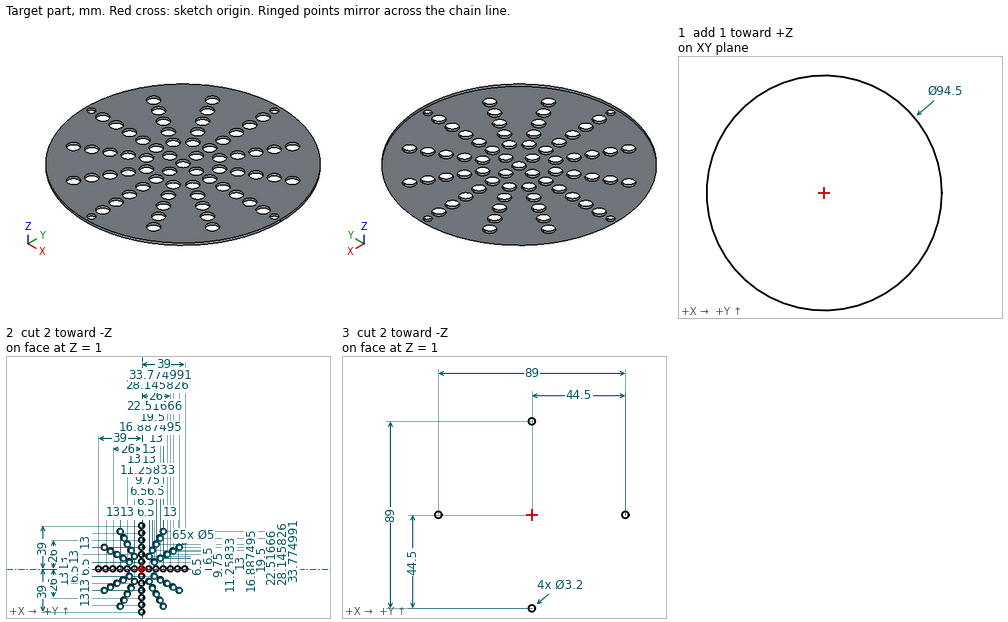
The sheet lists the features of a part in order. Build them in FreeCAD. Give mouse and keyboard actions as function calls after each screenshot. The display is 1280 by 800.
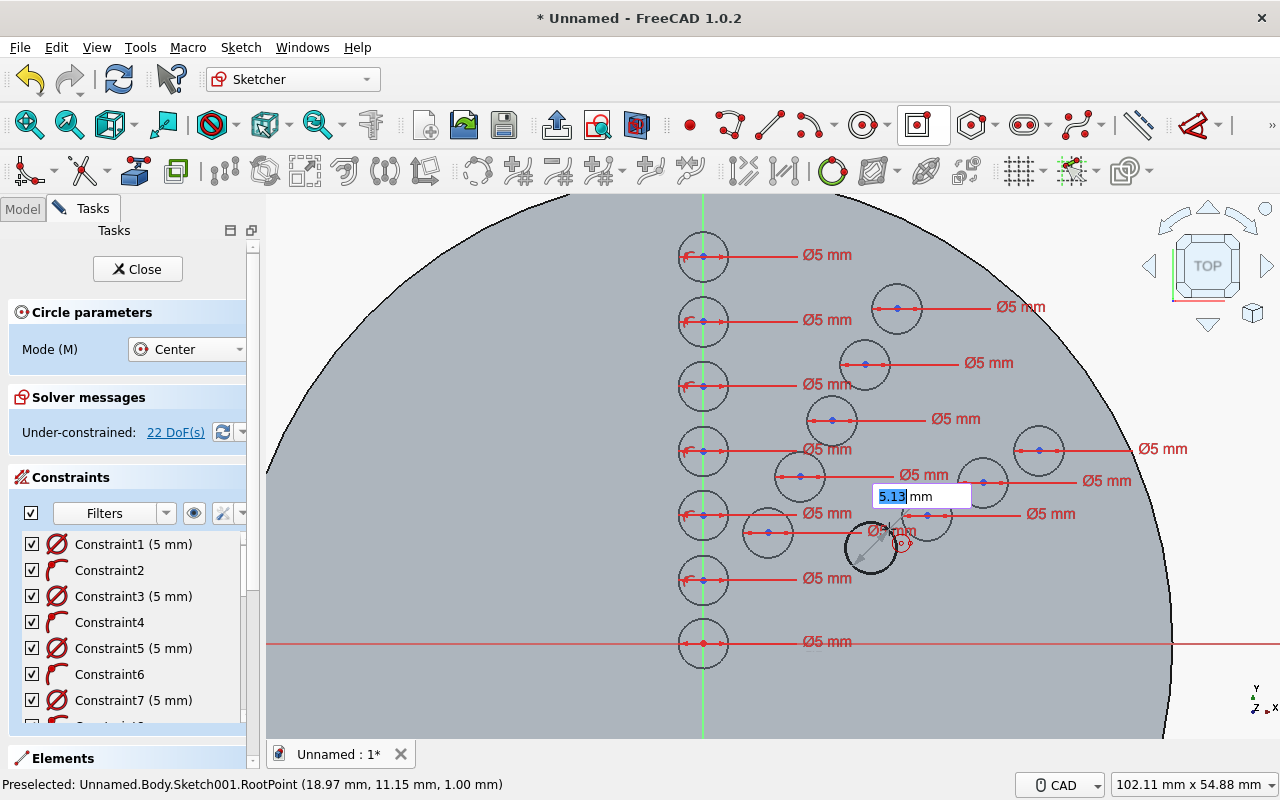
text(5)
key(Return)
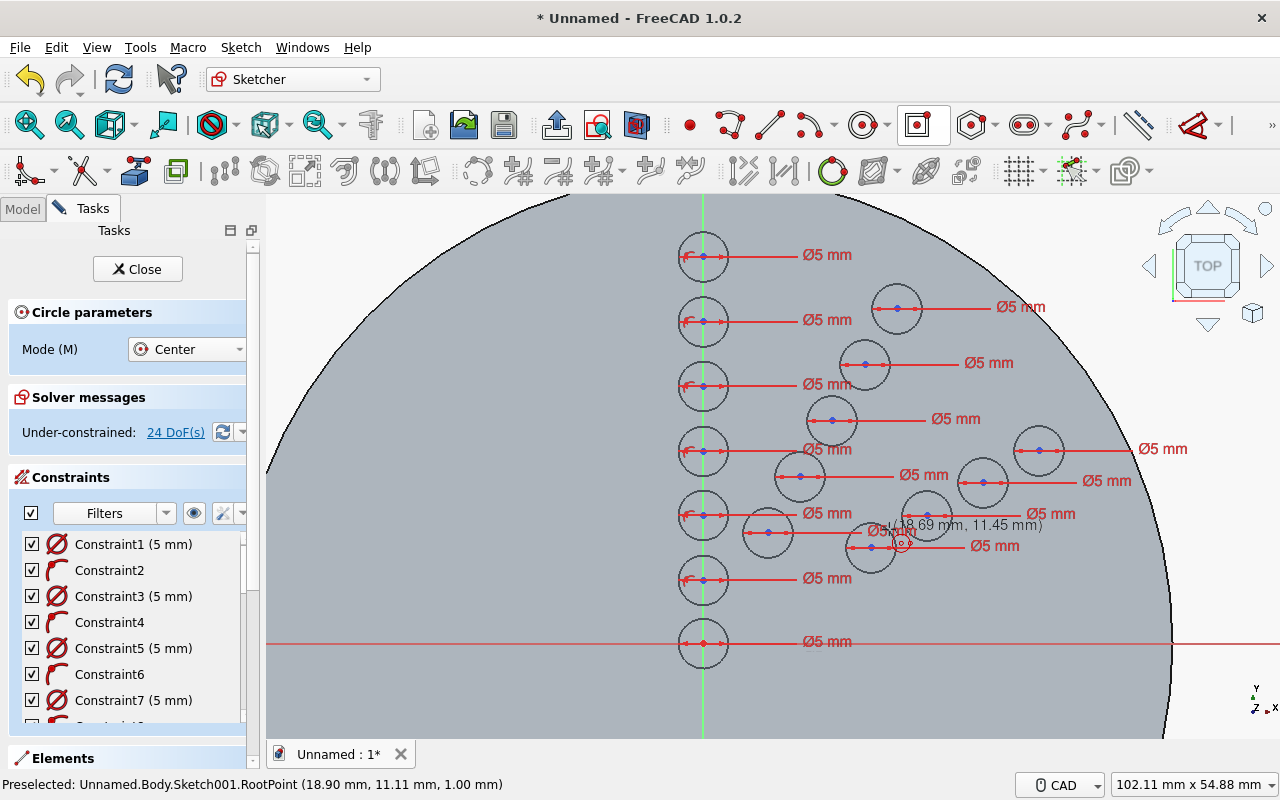
click(815, 579)
move(833, 562)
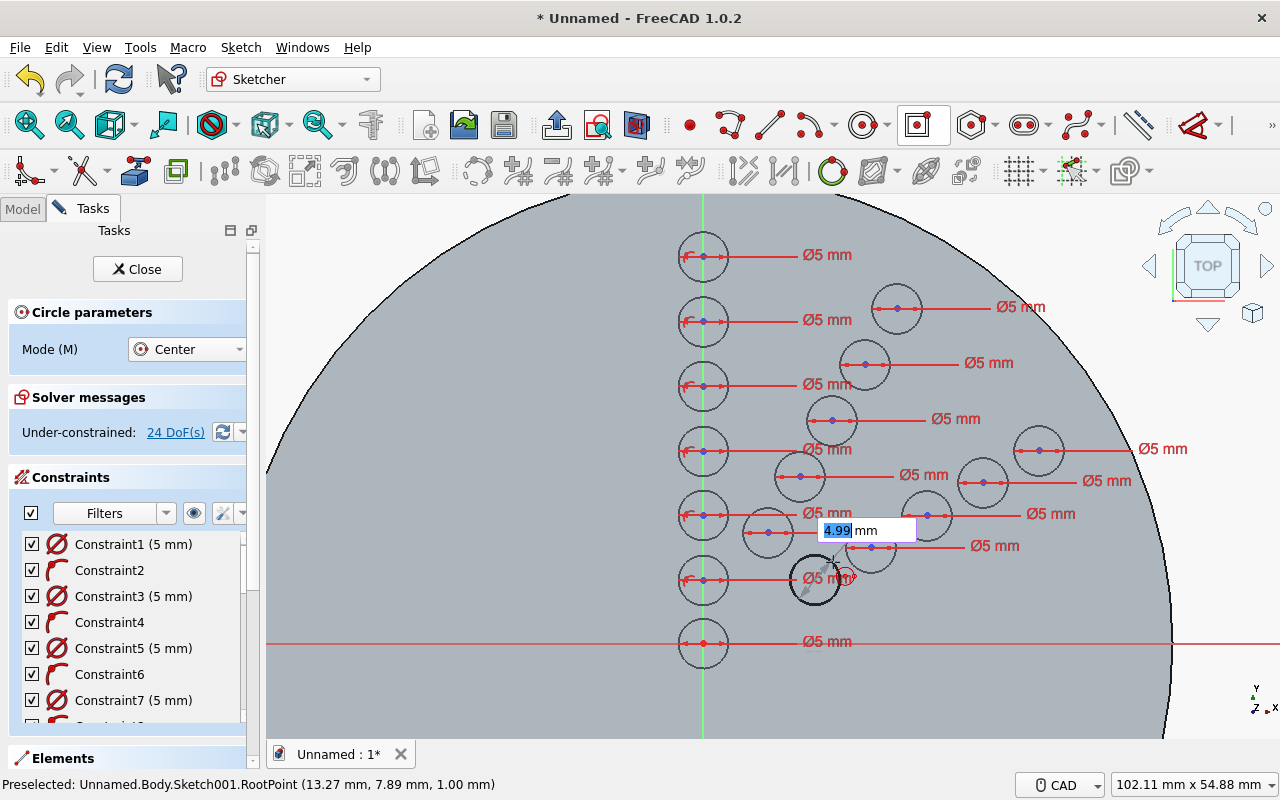
text(5)
key(Return)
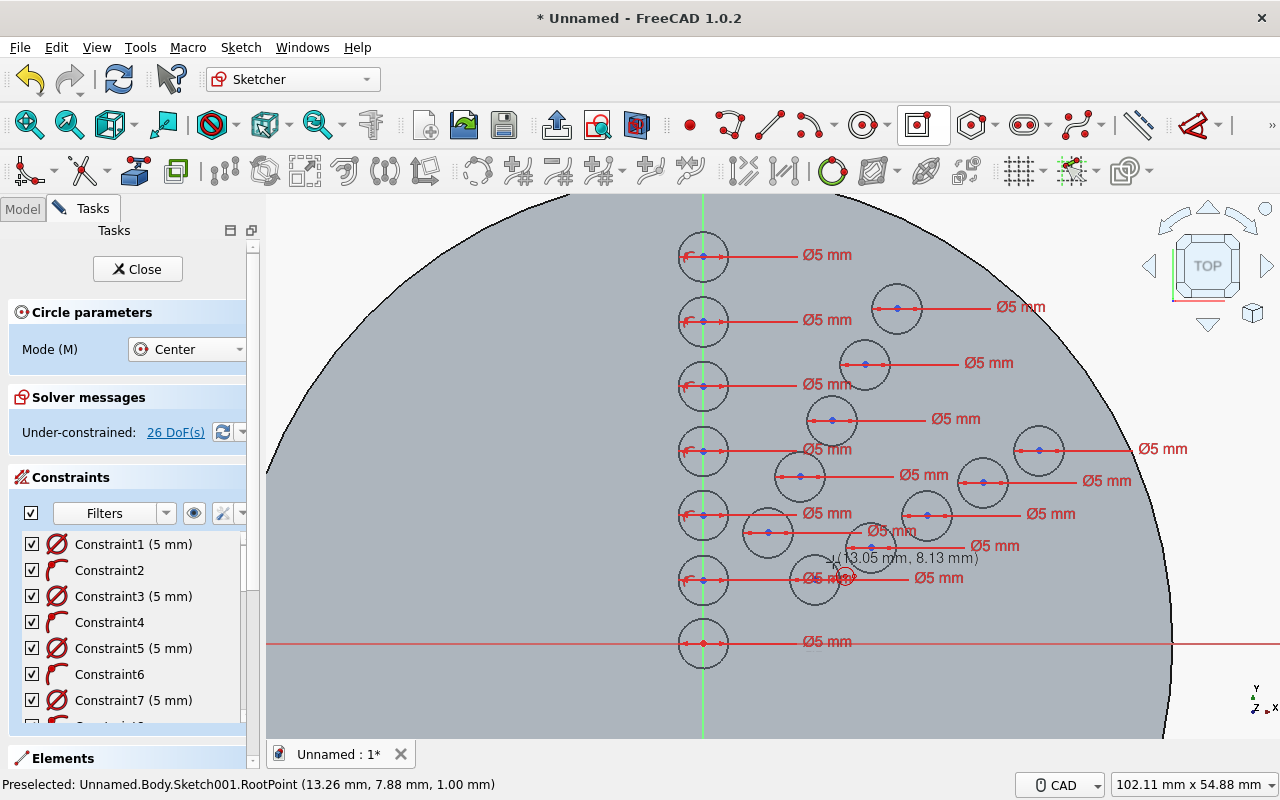
click(1091, 644)
move(1108, 626)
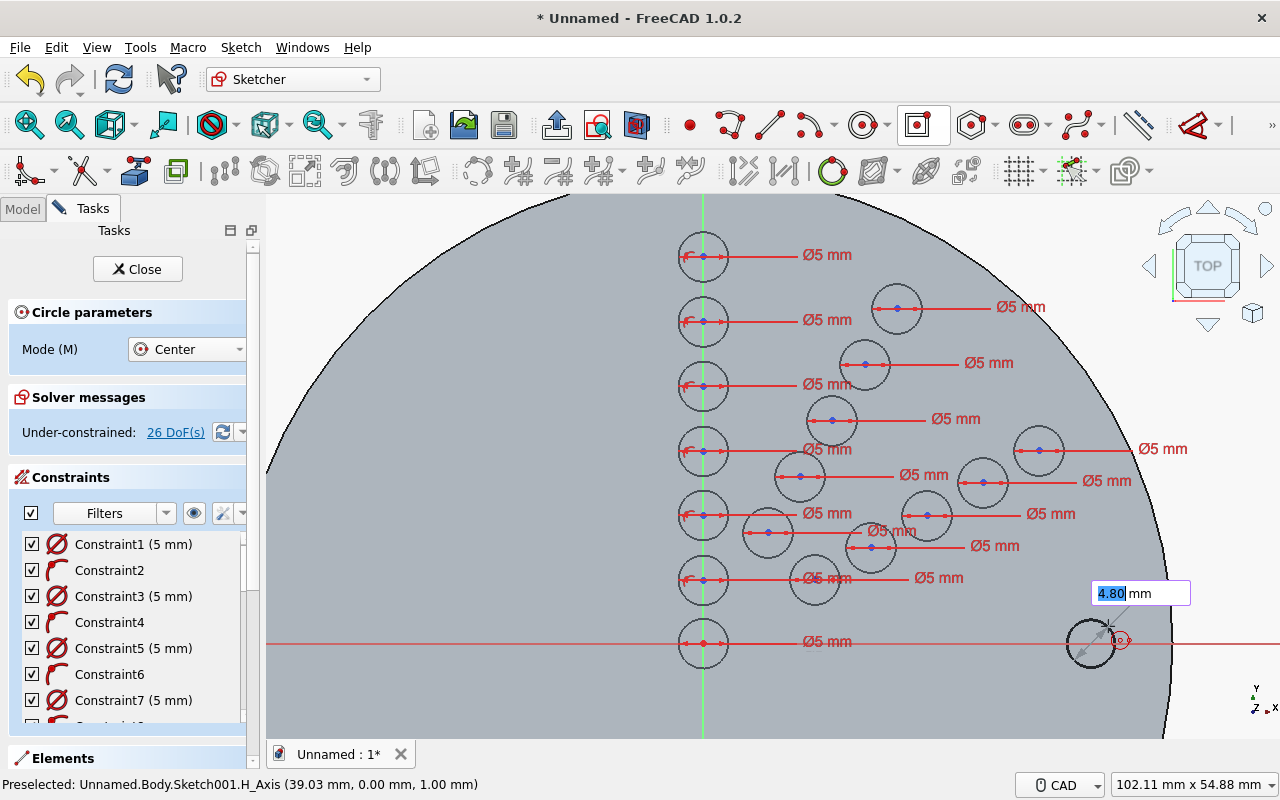
text(5)
key(Return)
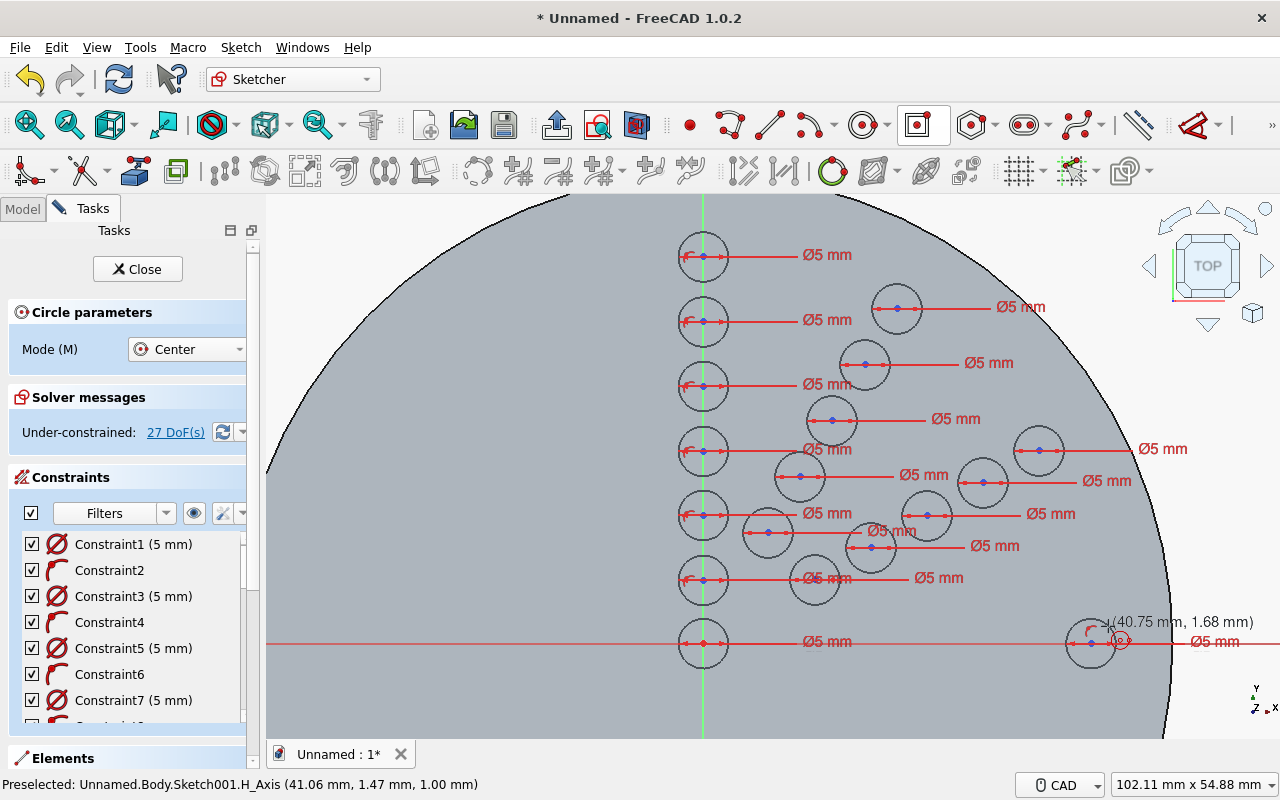
click(1026, 644)
move(1044, 626)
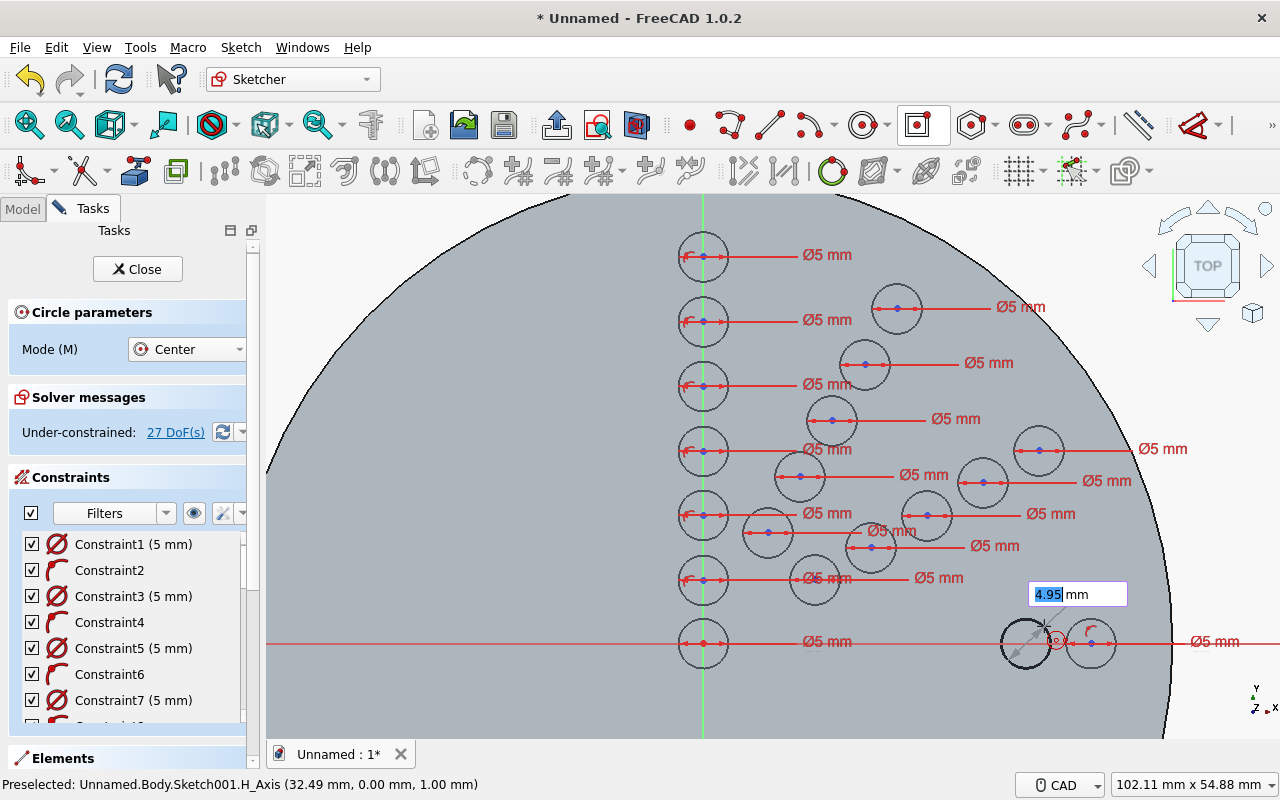
text(5)
key(Return)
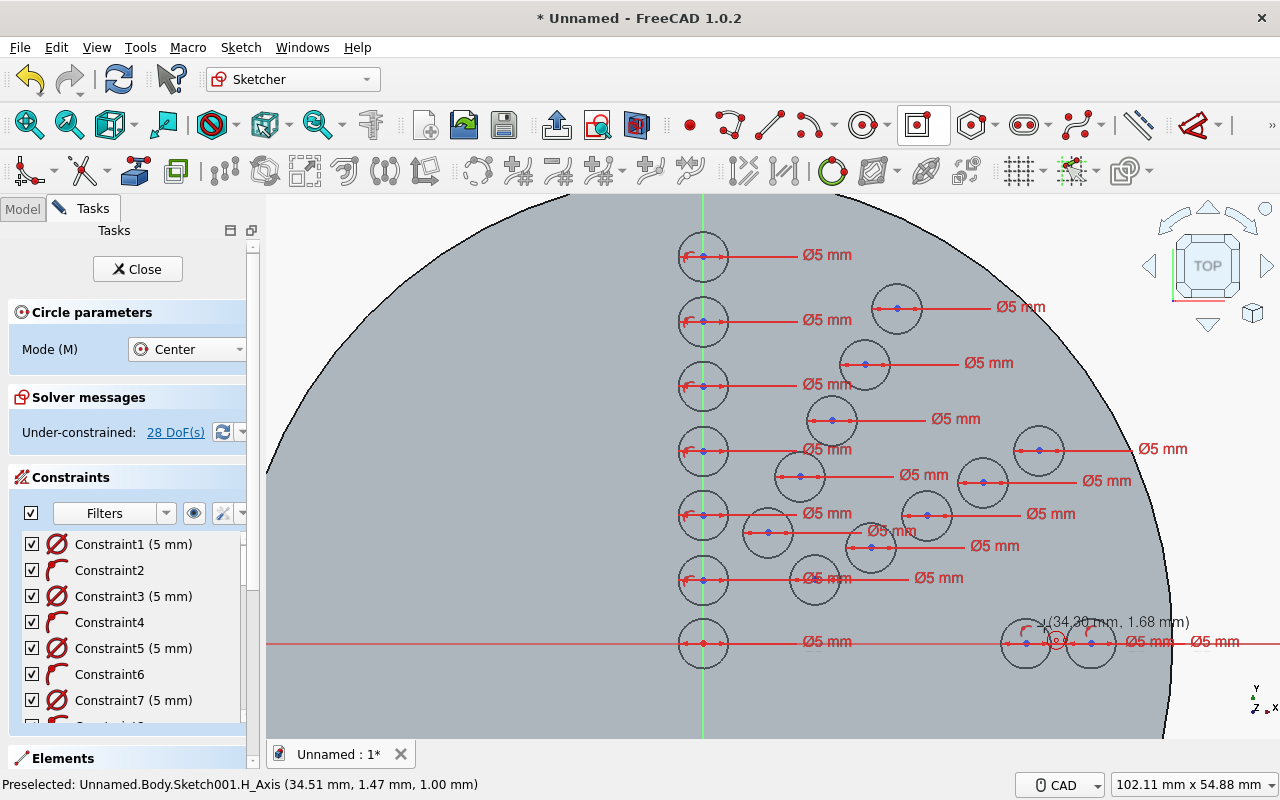
click(962, 644)
move(979, 626)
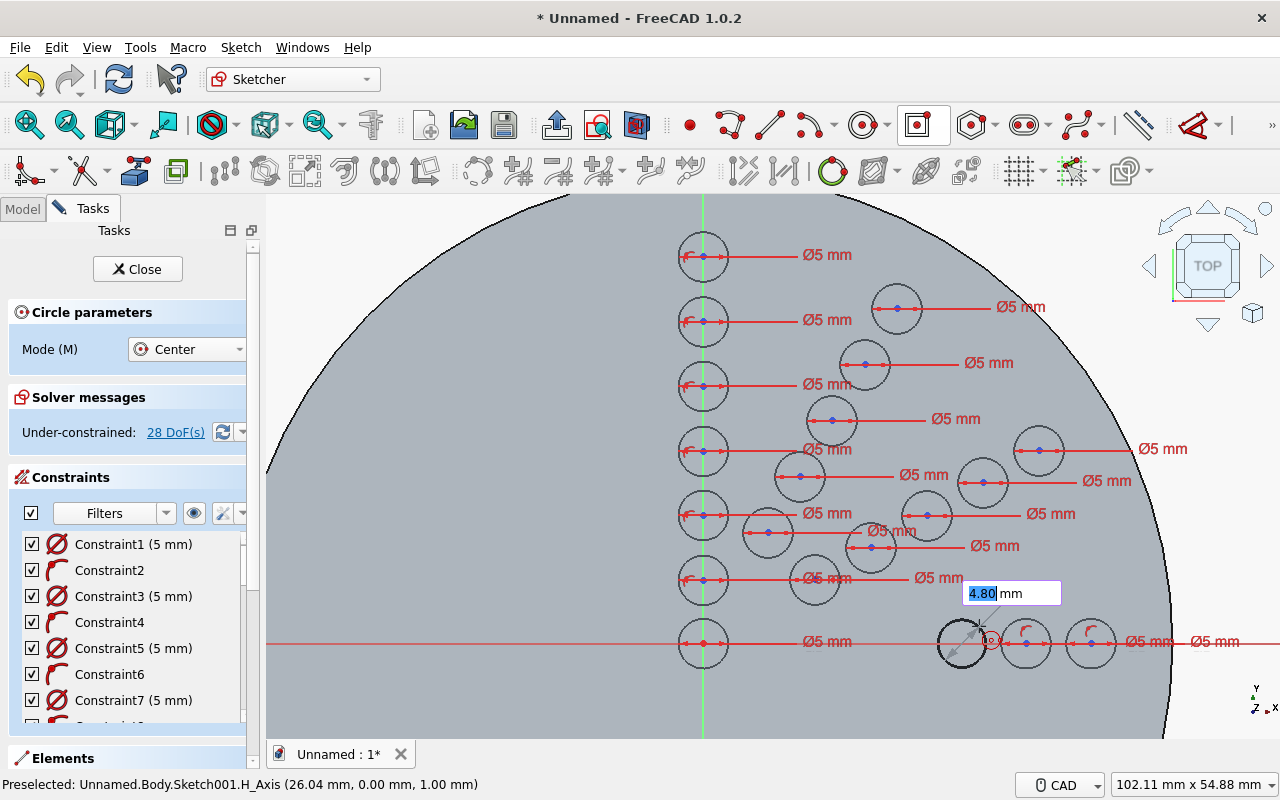
text(5)
key(Return)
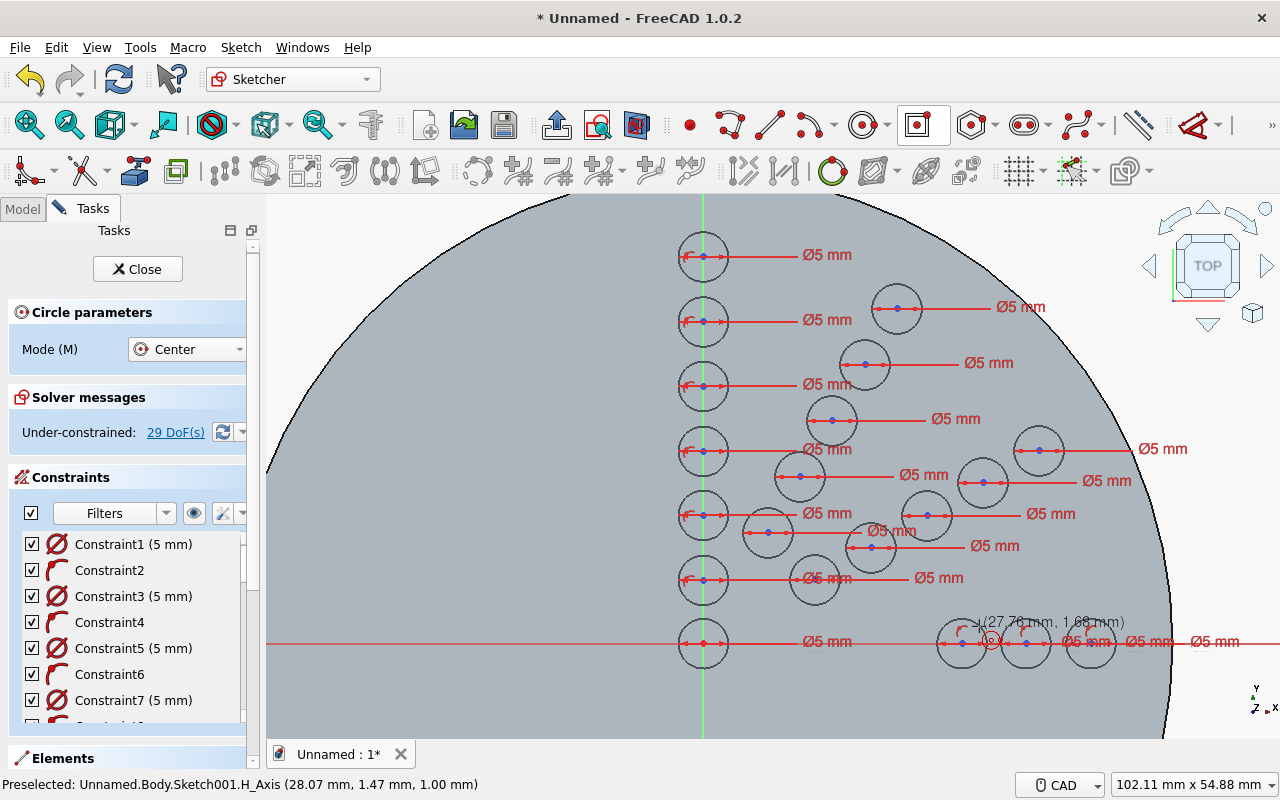
click(897, 644)
move(915, 626)